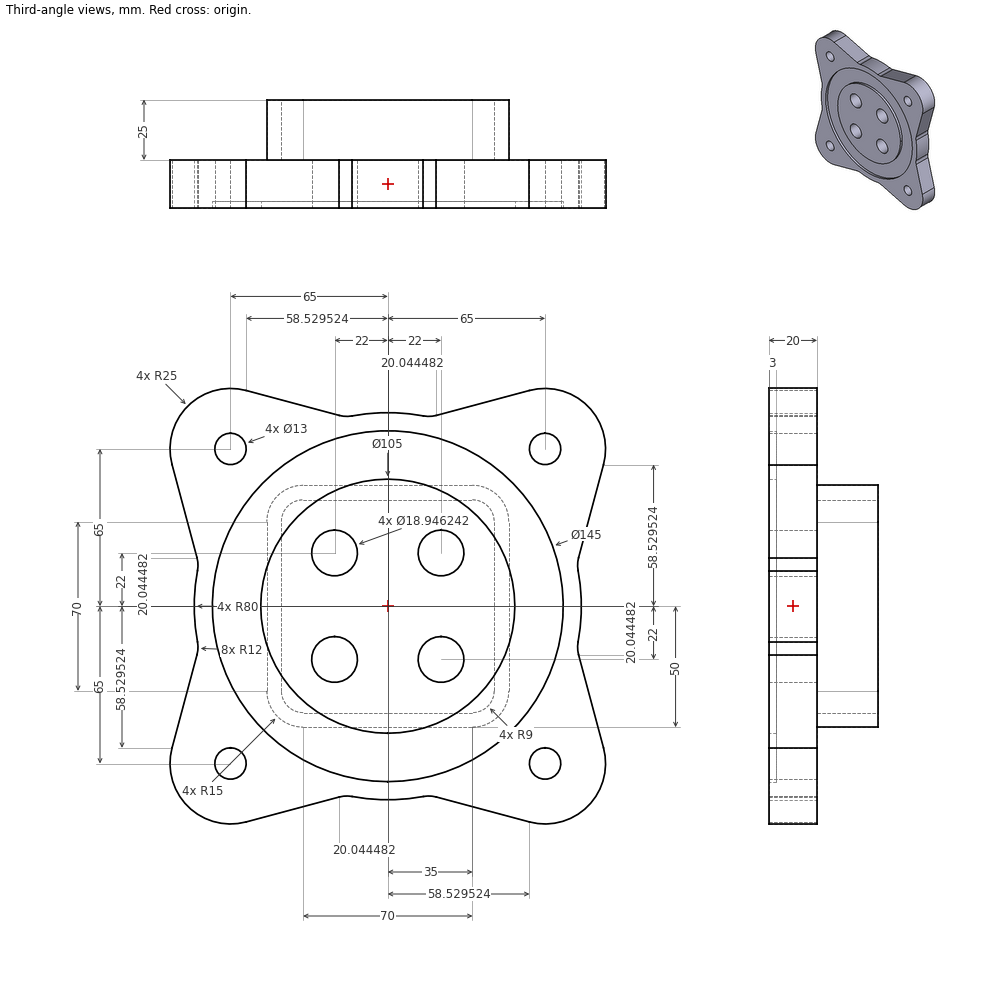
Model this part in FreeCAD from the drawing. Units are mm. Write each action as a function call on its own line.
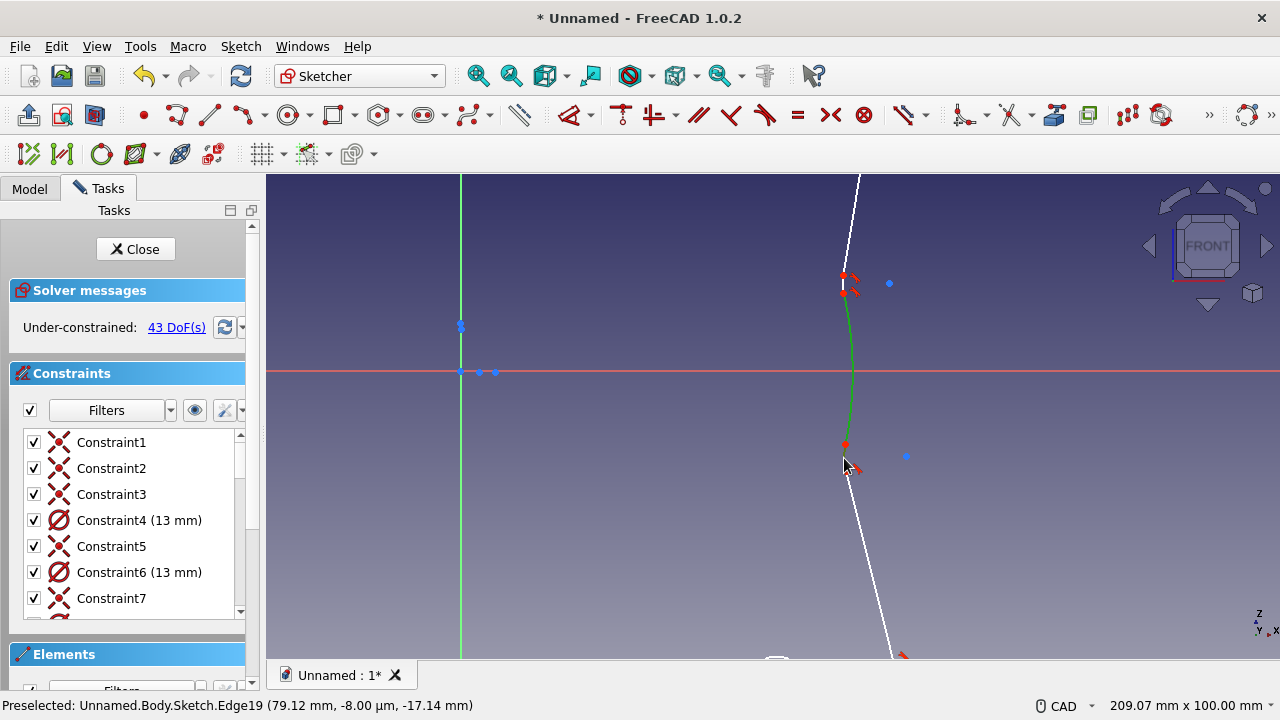
click(765, 116)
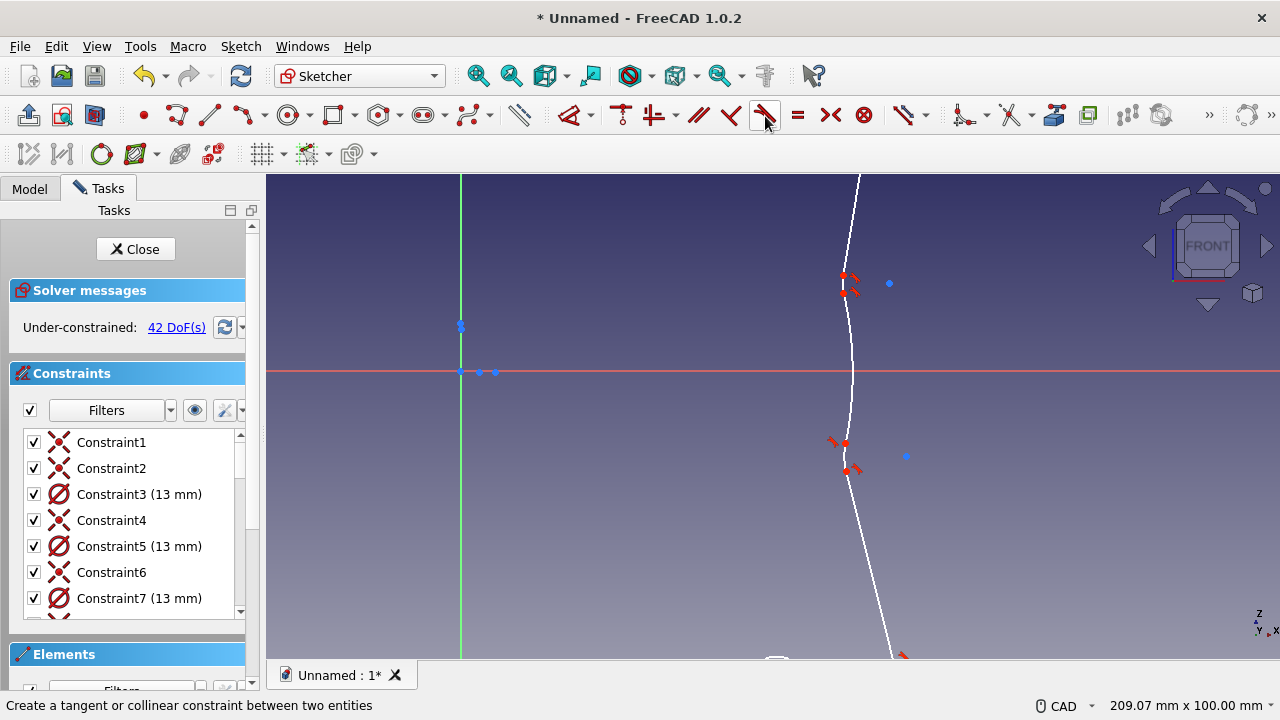
scroll(846, 443, down, 5)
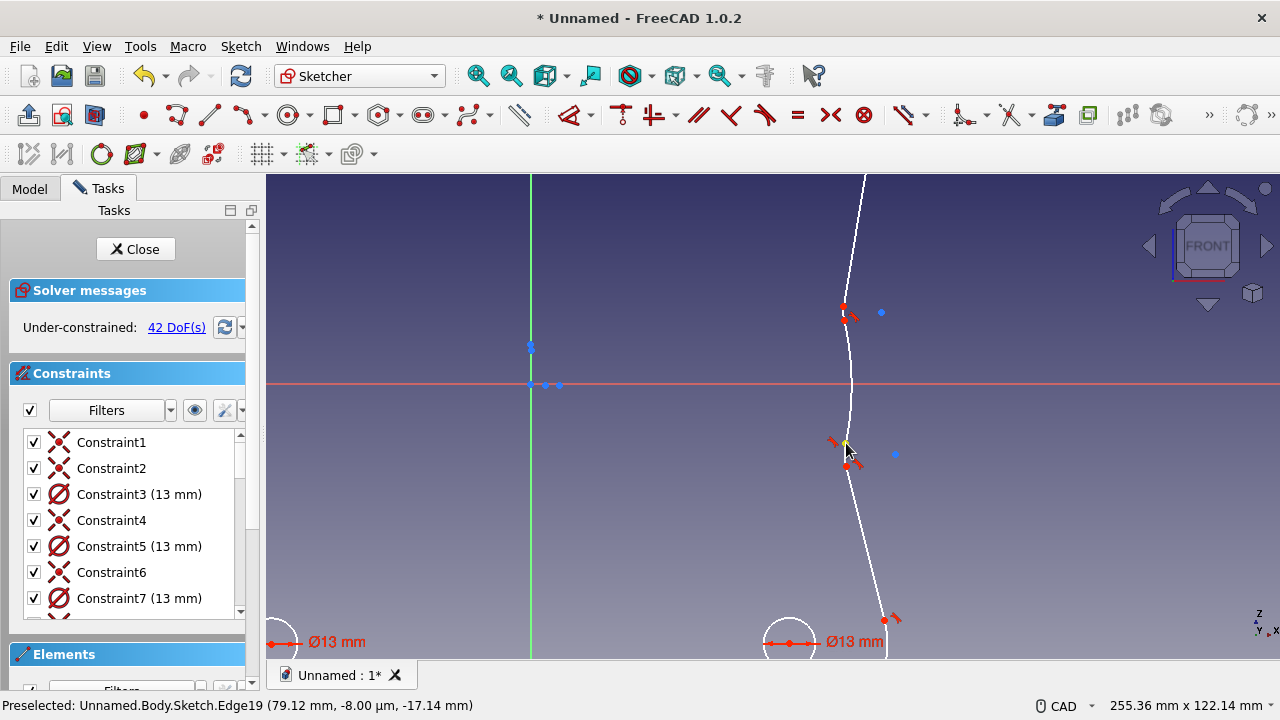
scroll(736, 556, up, 6)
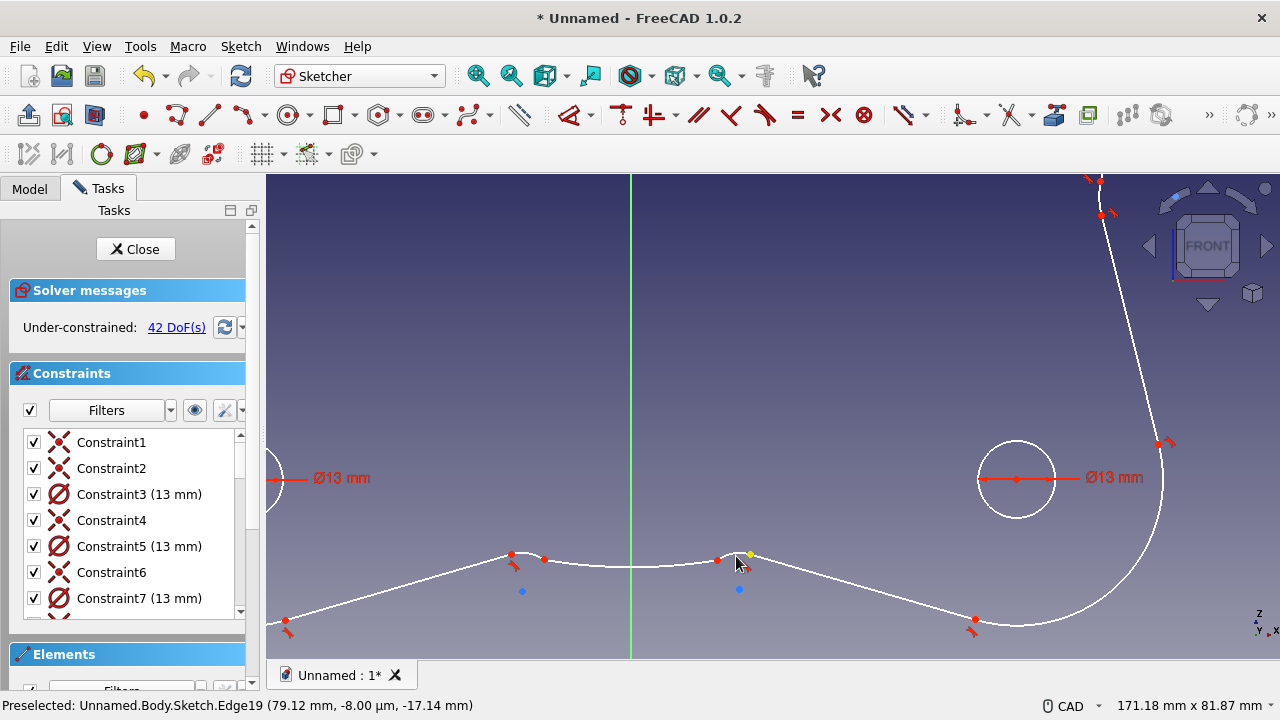
click(733, 553)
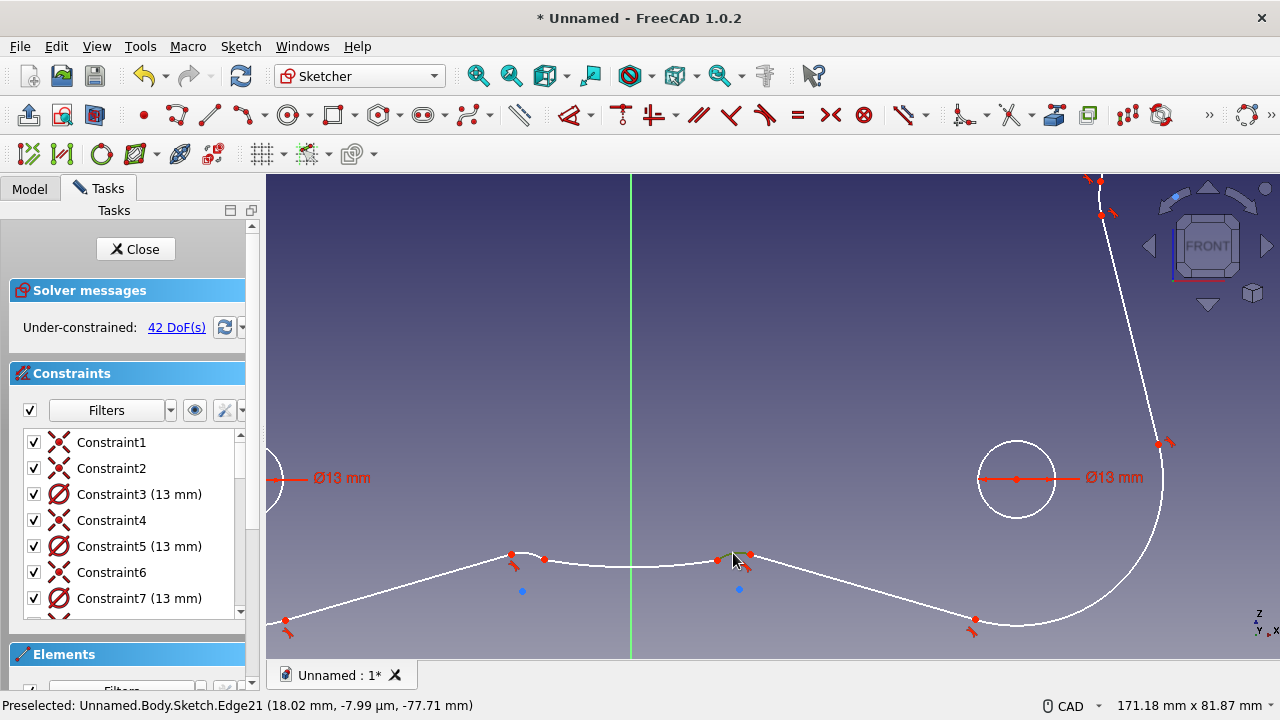
click(596, 566)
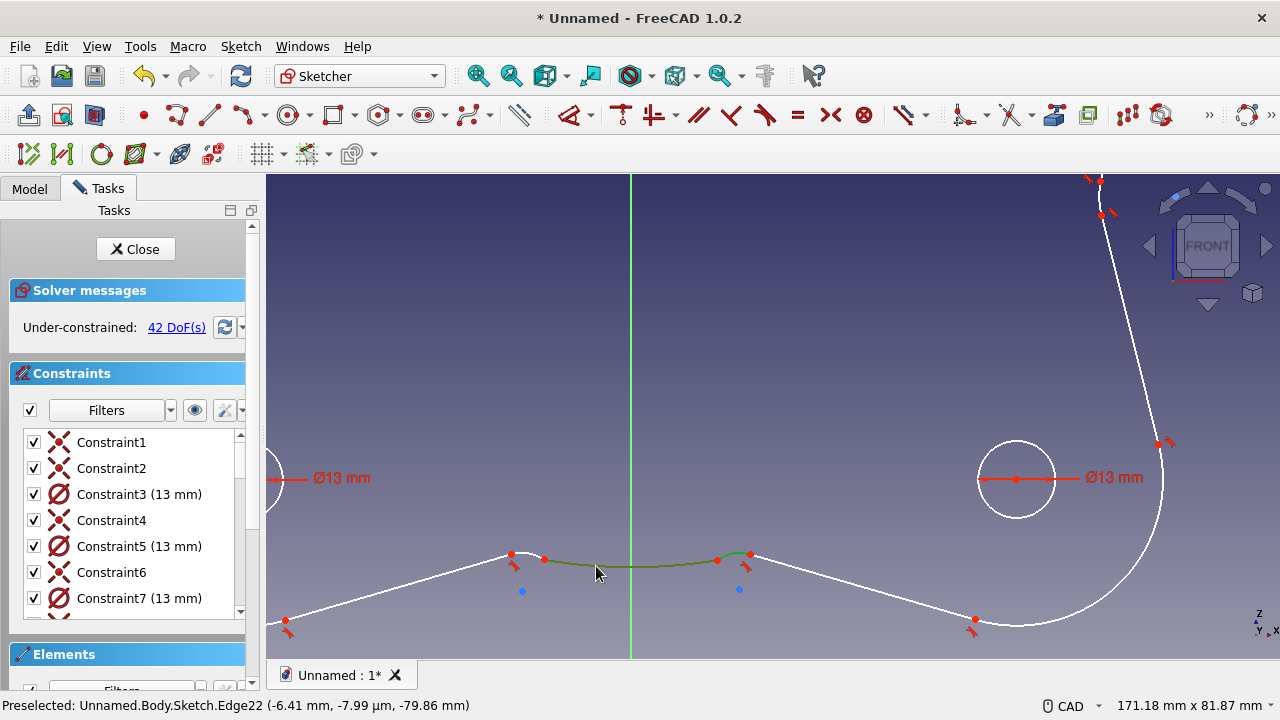
key(t)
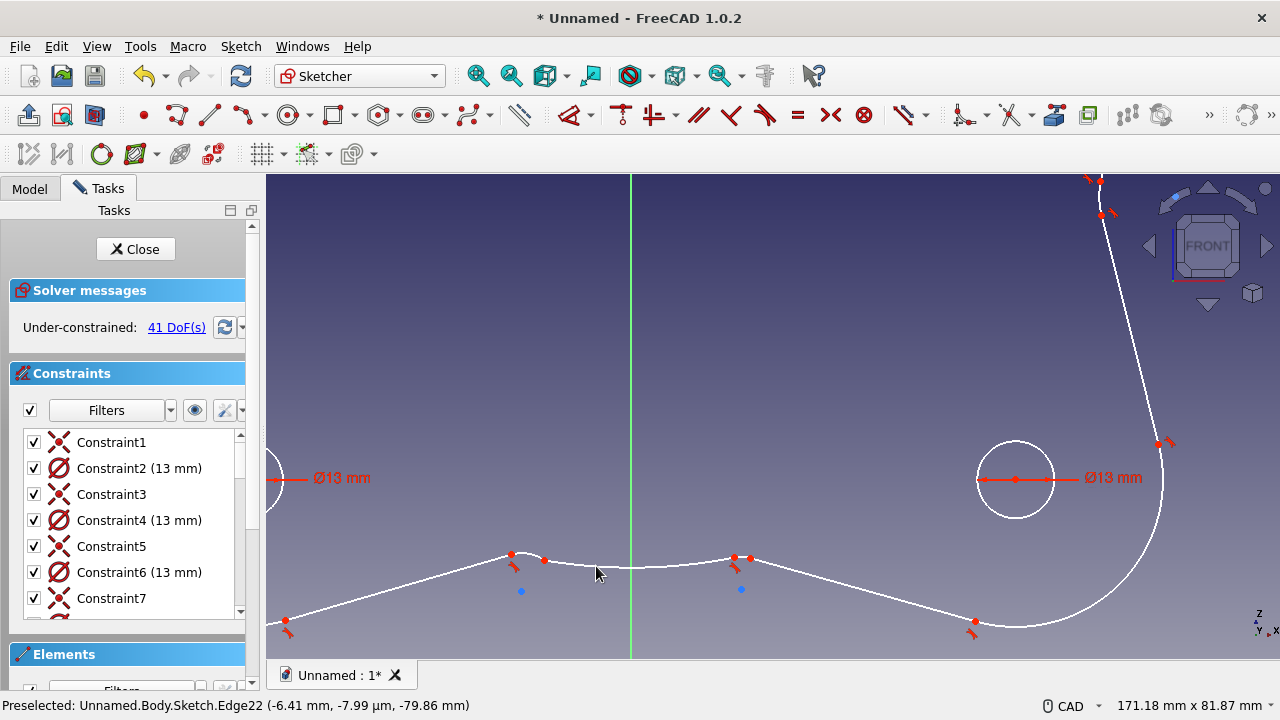
click(601, 567)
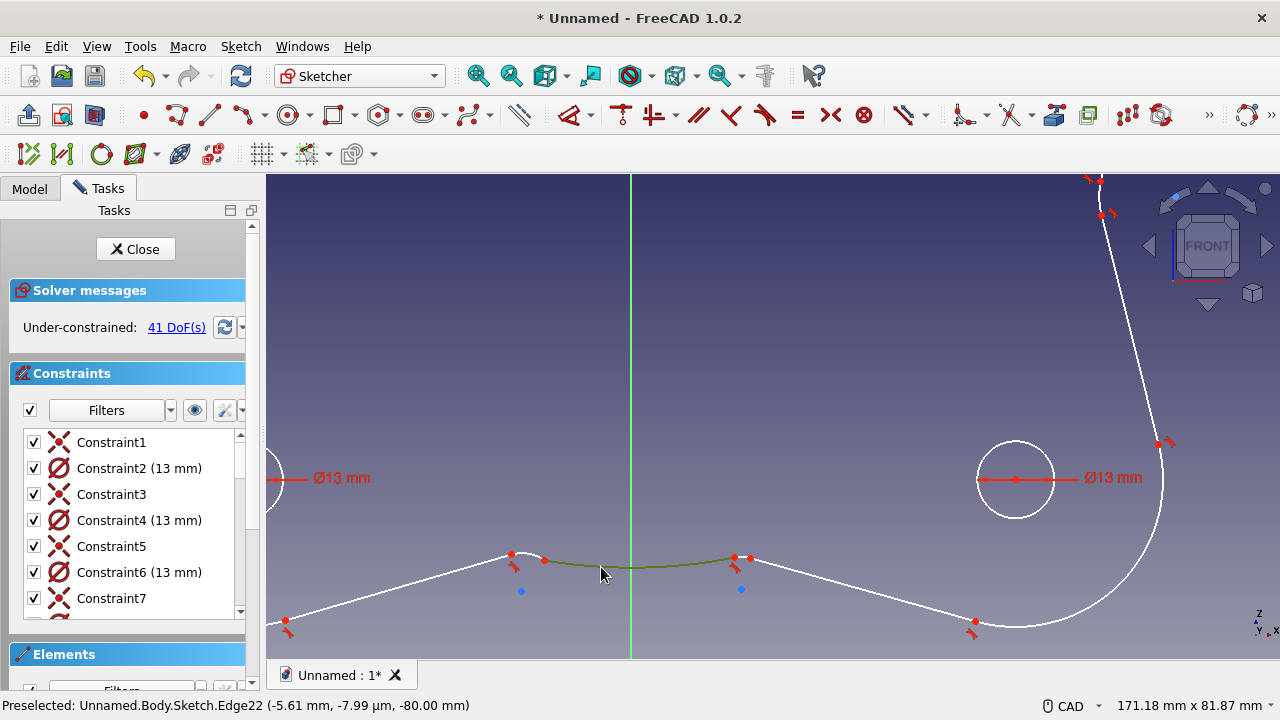
scroll(535, 555, up, 2)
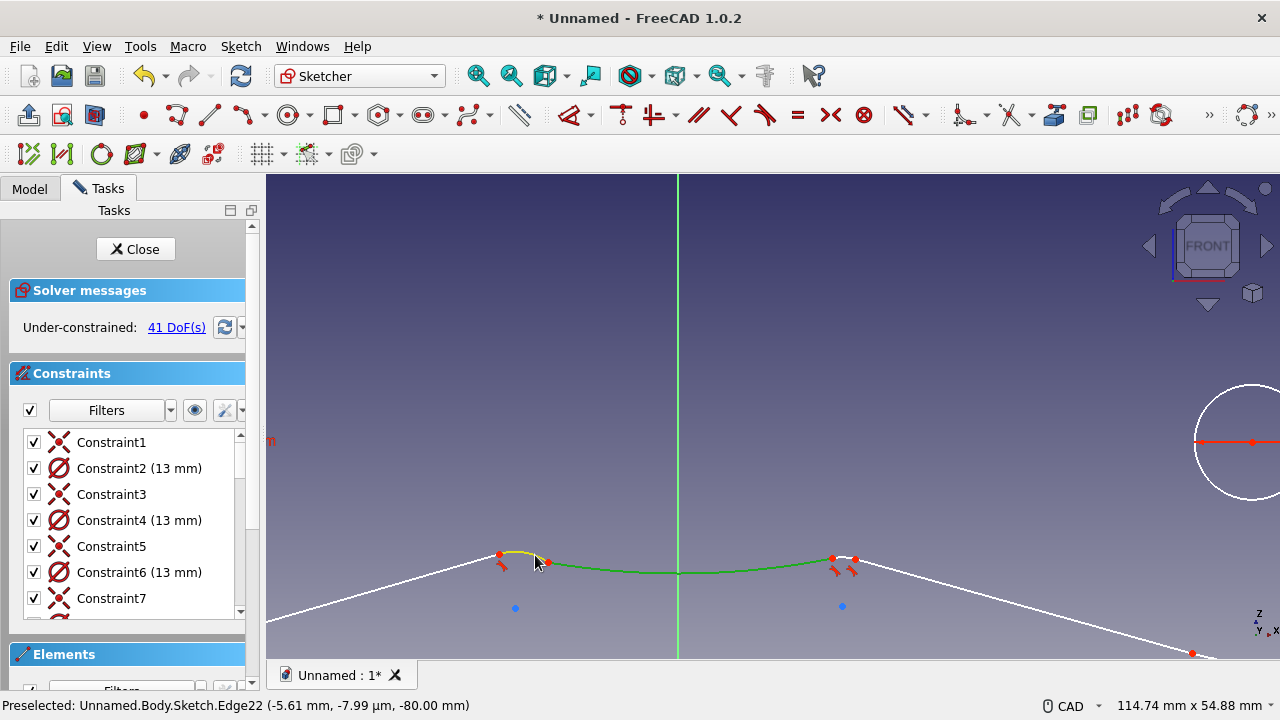
click(535, 555)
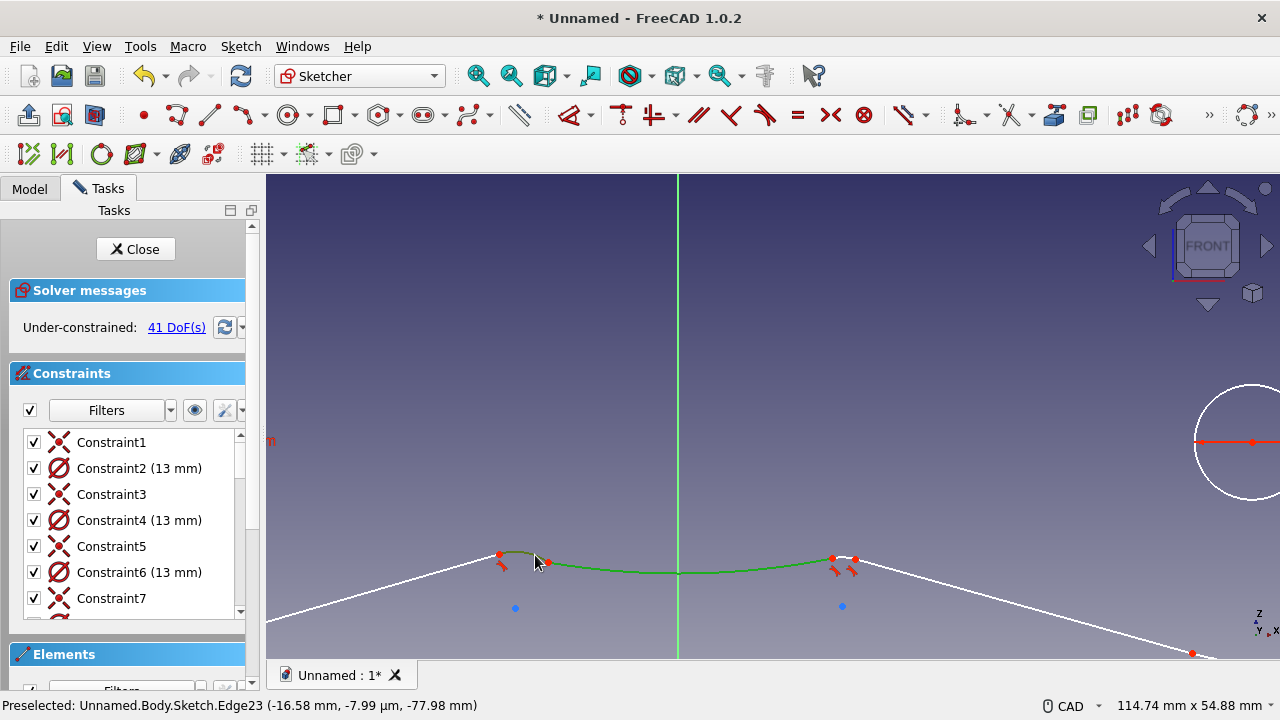
click(765, 116)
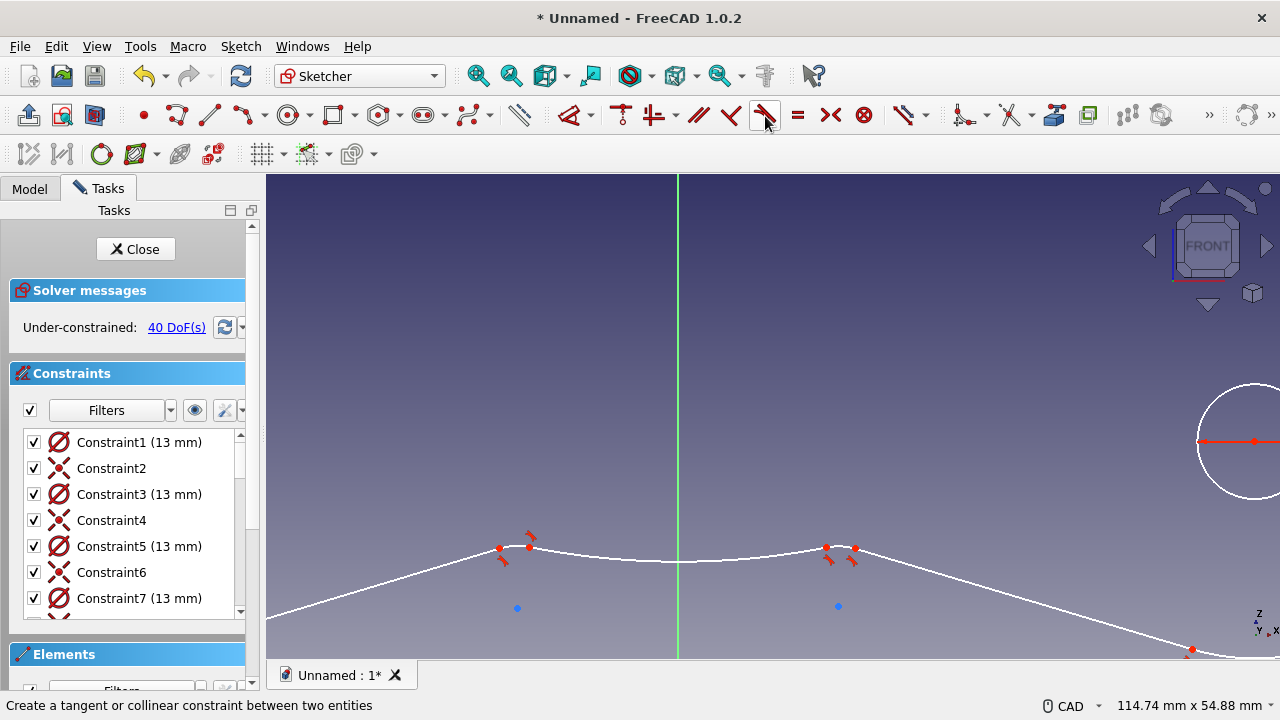
scroll(711, 556, down, 8)